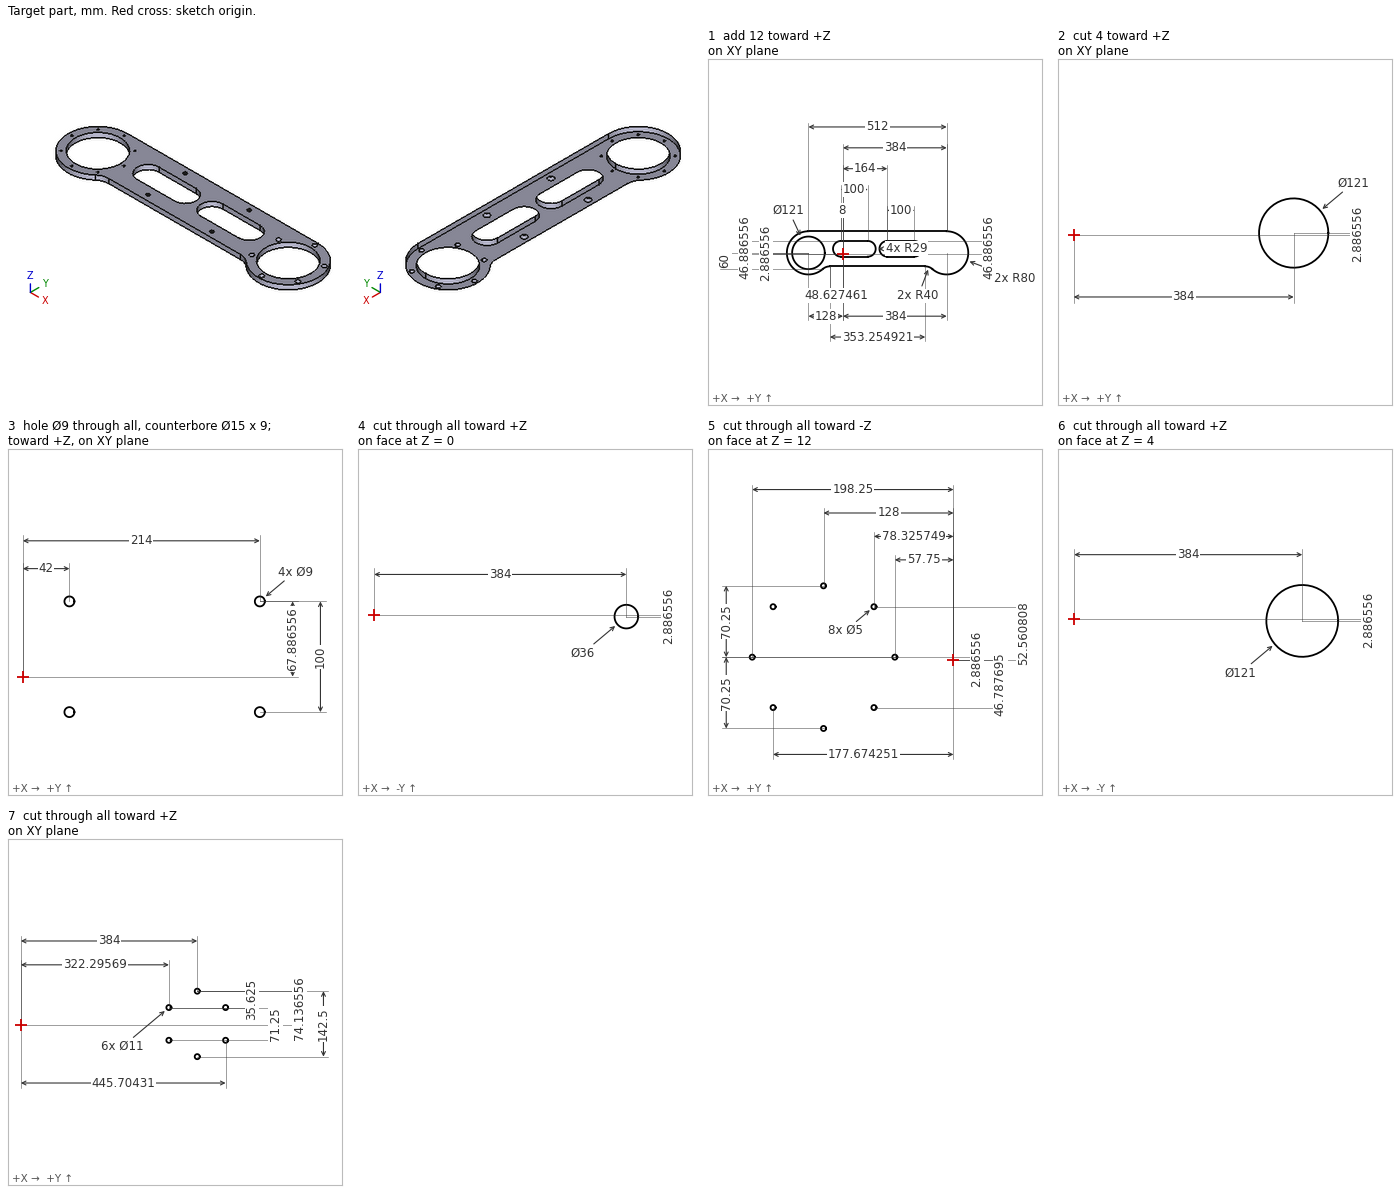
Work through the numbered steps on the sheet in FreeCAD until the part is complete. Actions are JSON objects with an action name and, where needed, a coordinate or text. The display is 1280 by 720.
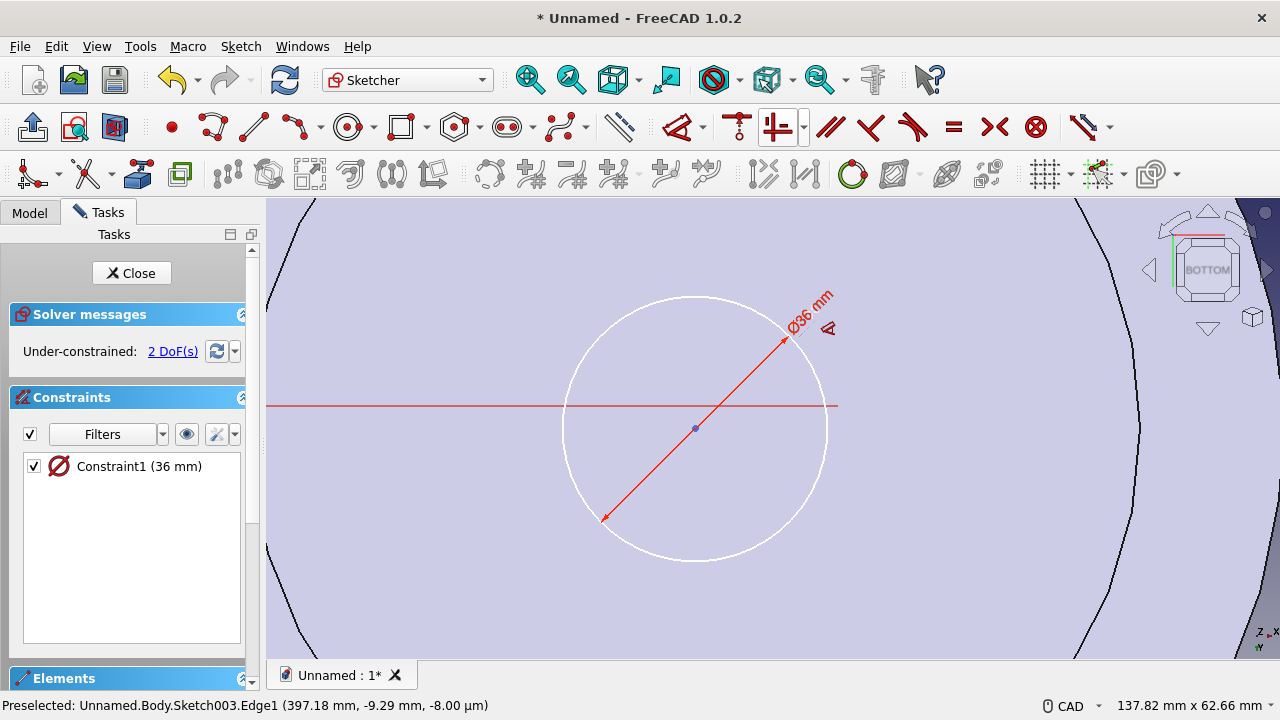
{"action": "left_click", "coordinate": [695, 429]}
{"action": "left_click", "coordinate": [495, 372]}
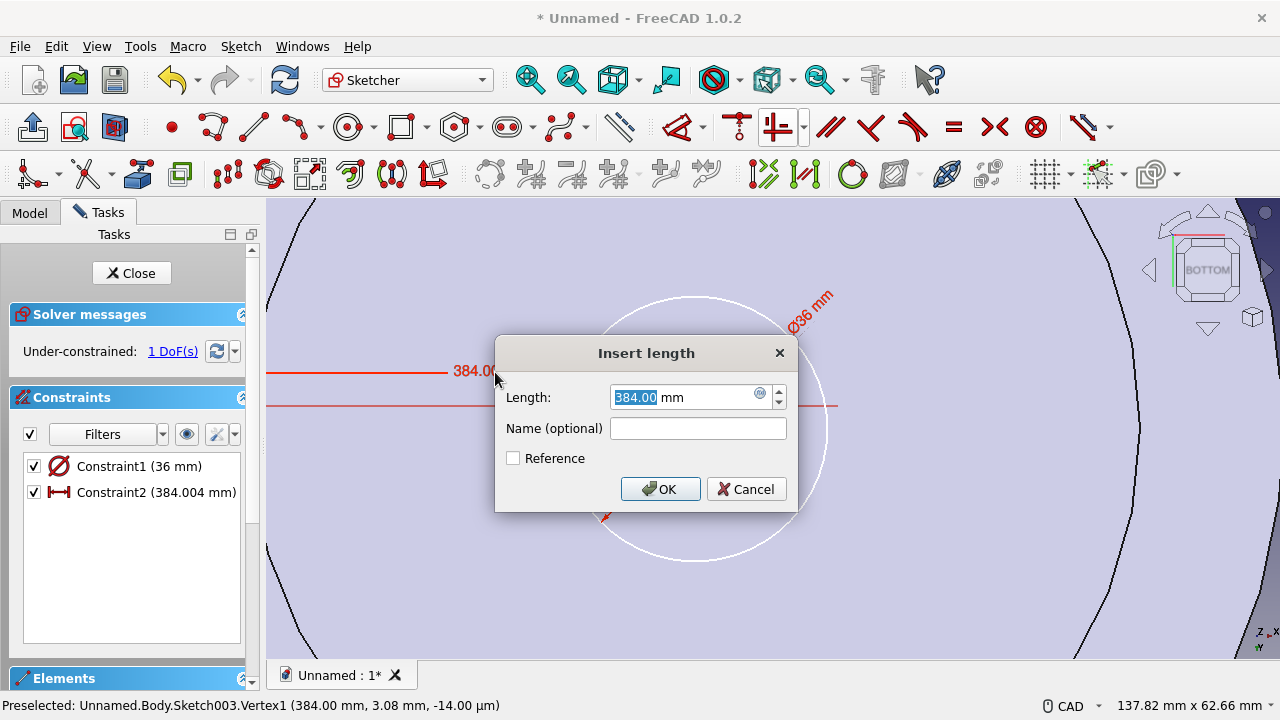
{"action": "type", "text": "384"}
{"action": "key", "text": "Return"}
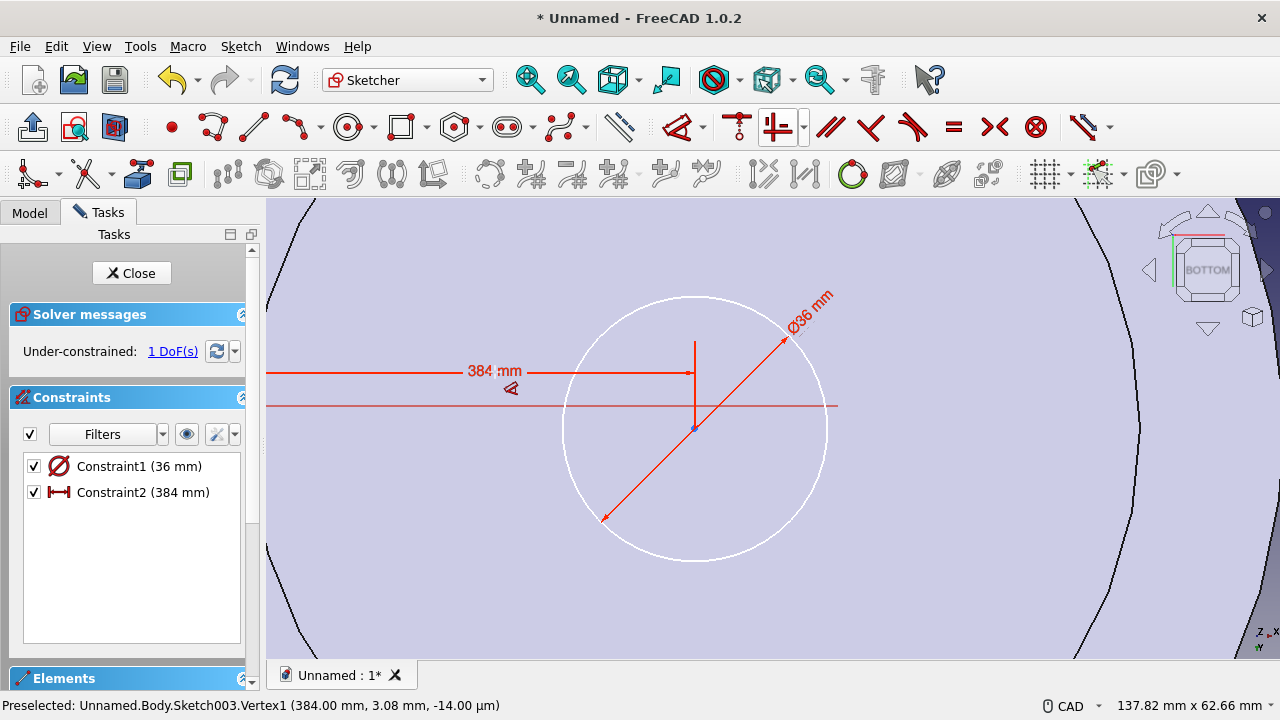
{"action": "scroll", "coordinate": [695, 429], "scroll_direction": "up", "scroll_amount": 4}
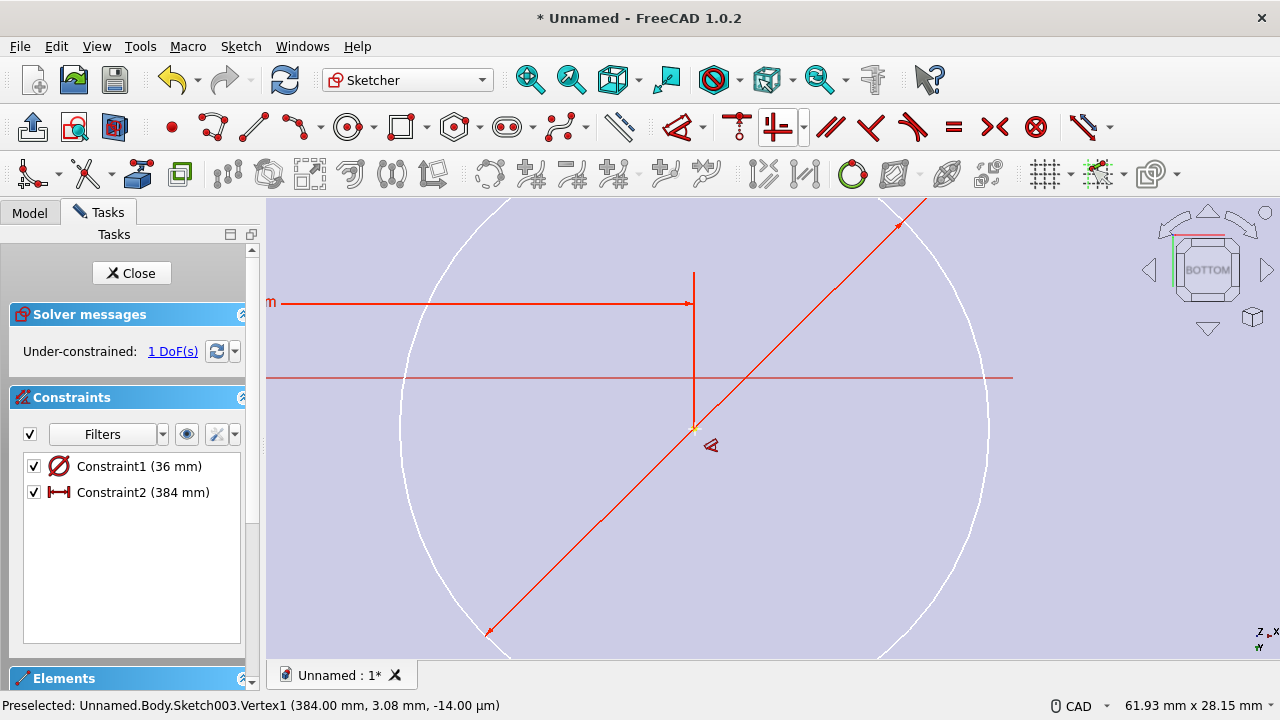
{"action": "left_click", "coordinate": [694, 428]}
{"action": "left_click", "coordinate": [728, 403]}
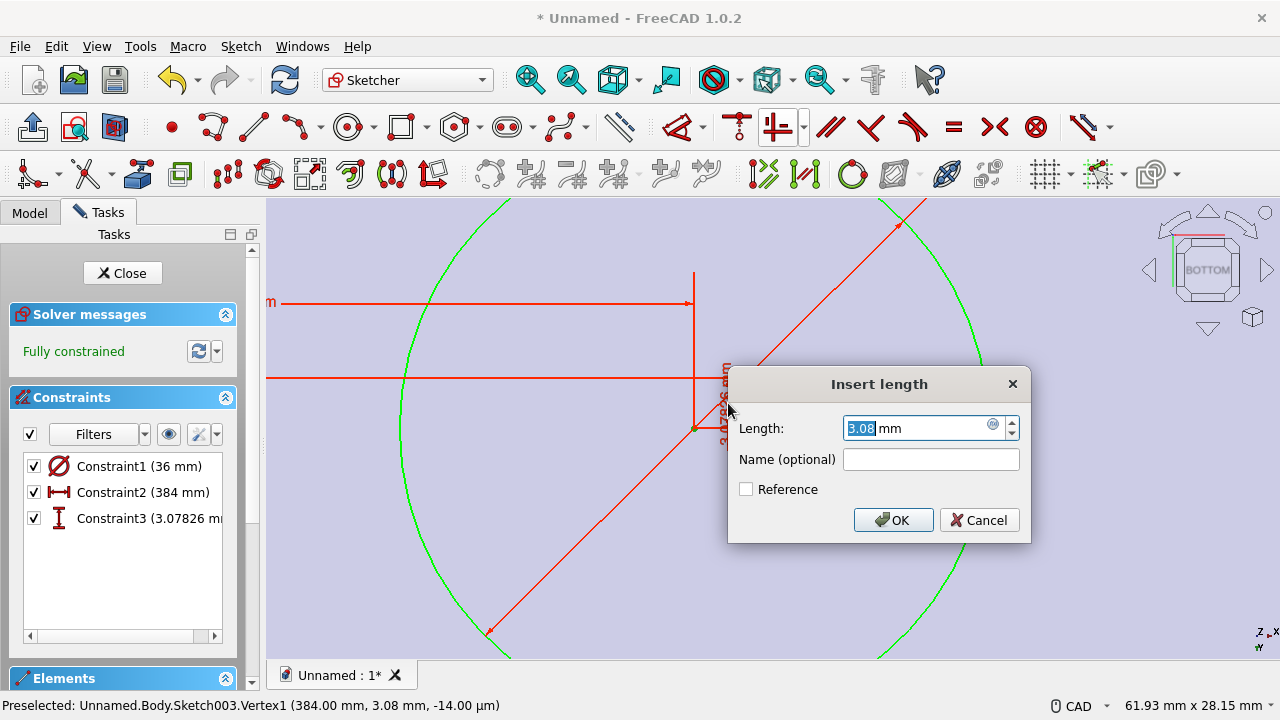
{"action": "type", "text": "2.886556"}
{"action": "key", "text": "Return"}
{"action": "key", "text": "Escape"}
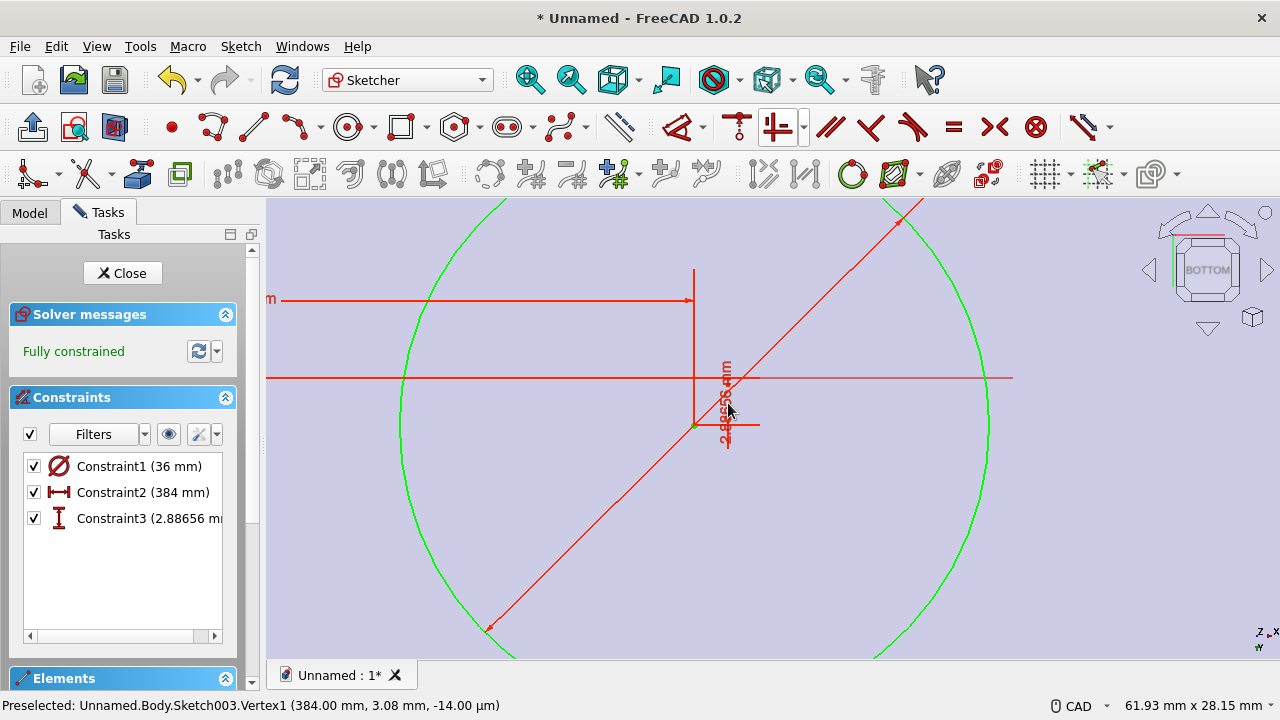
{"action": "left_click", "coordinate": [123, 273]}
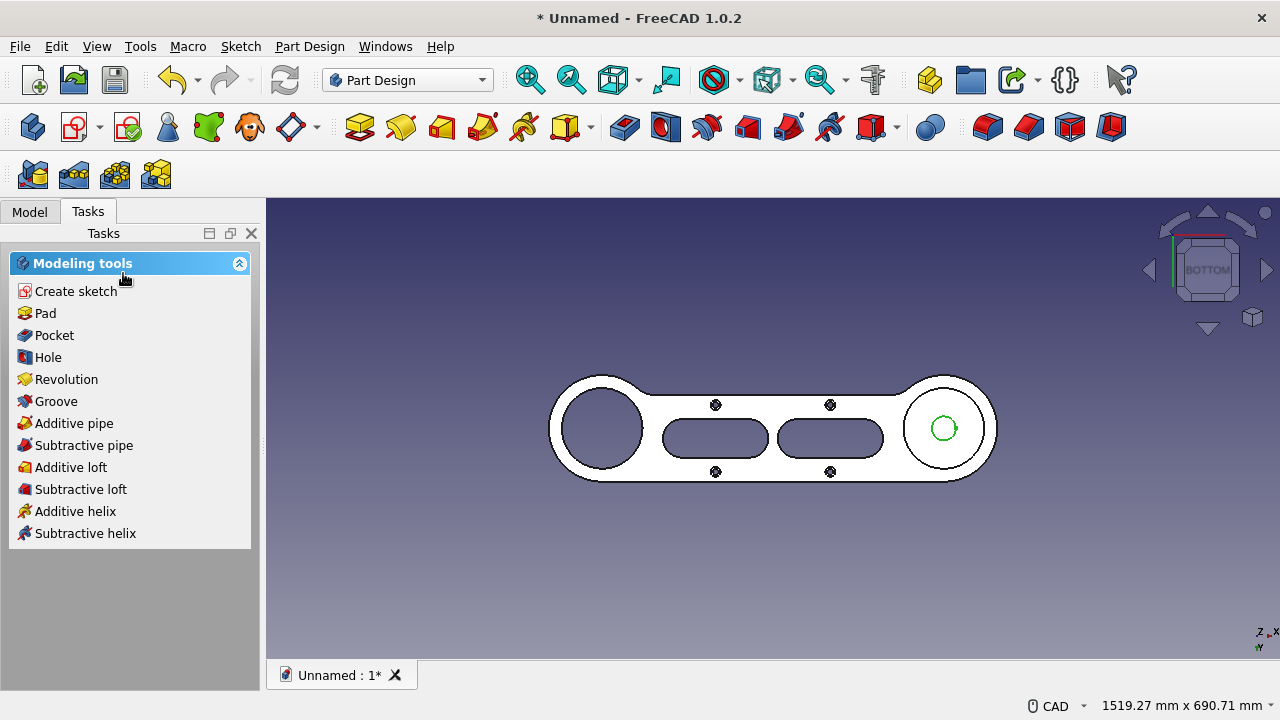
{"action": "left_click", "coordinate": [625, 128]}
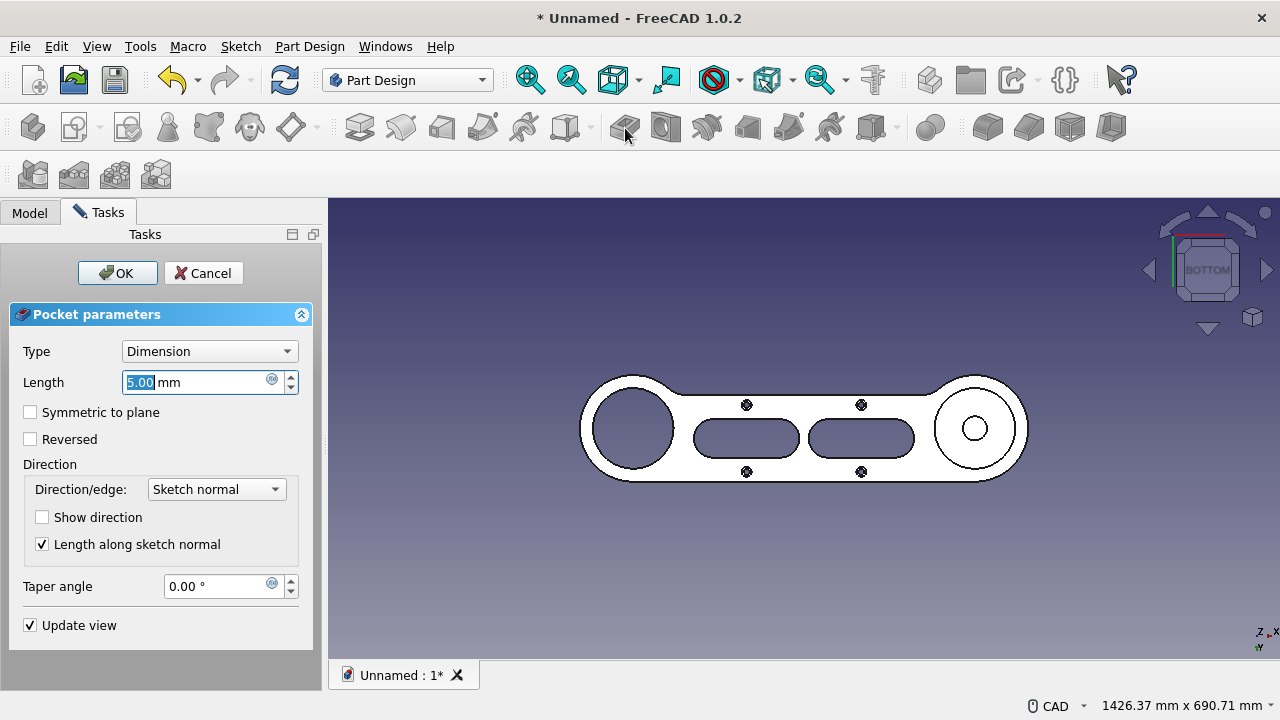
{"action": "left_click", "coordinate": [210, 352]}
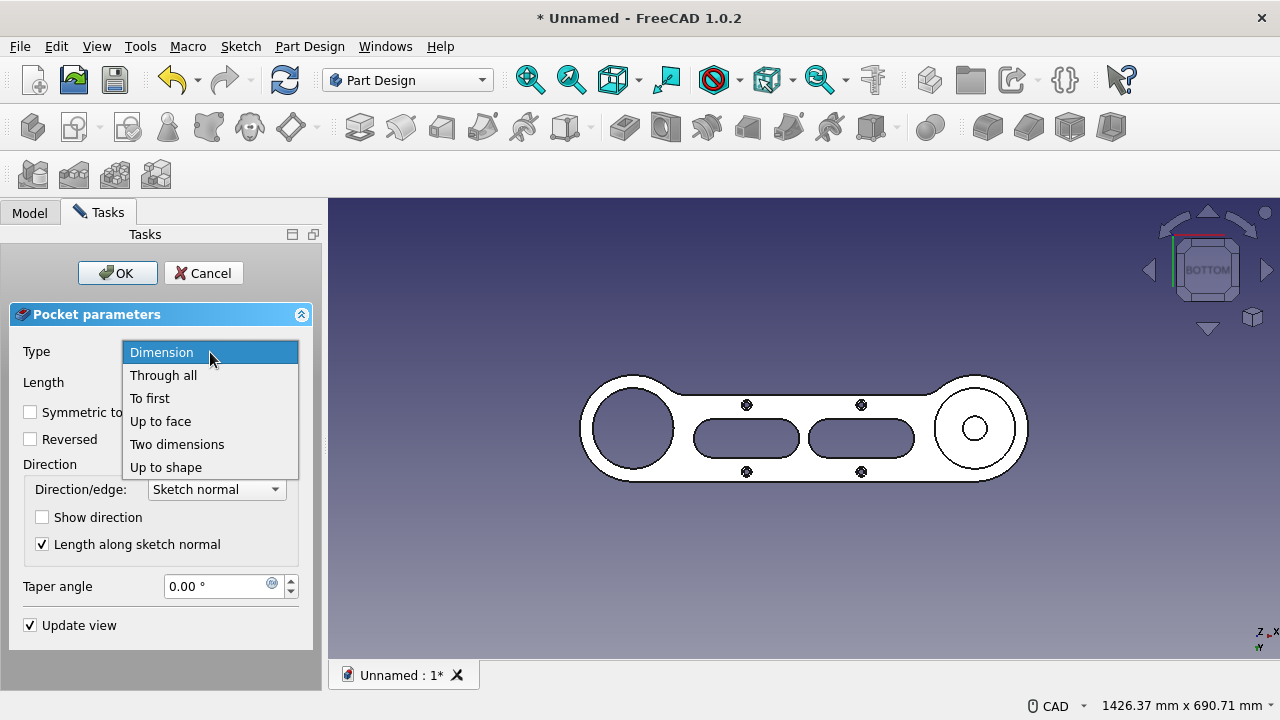
{"action": "left_click", "coordinate": [208, 376]}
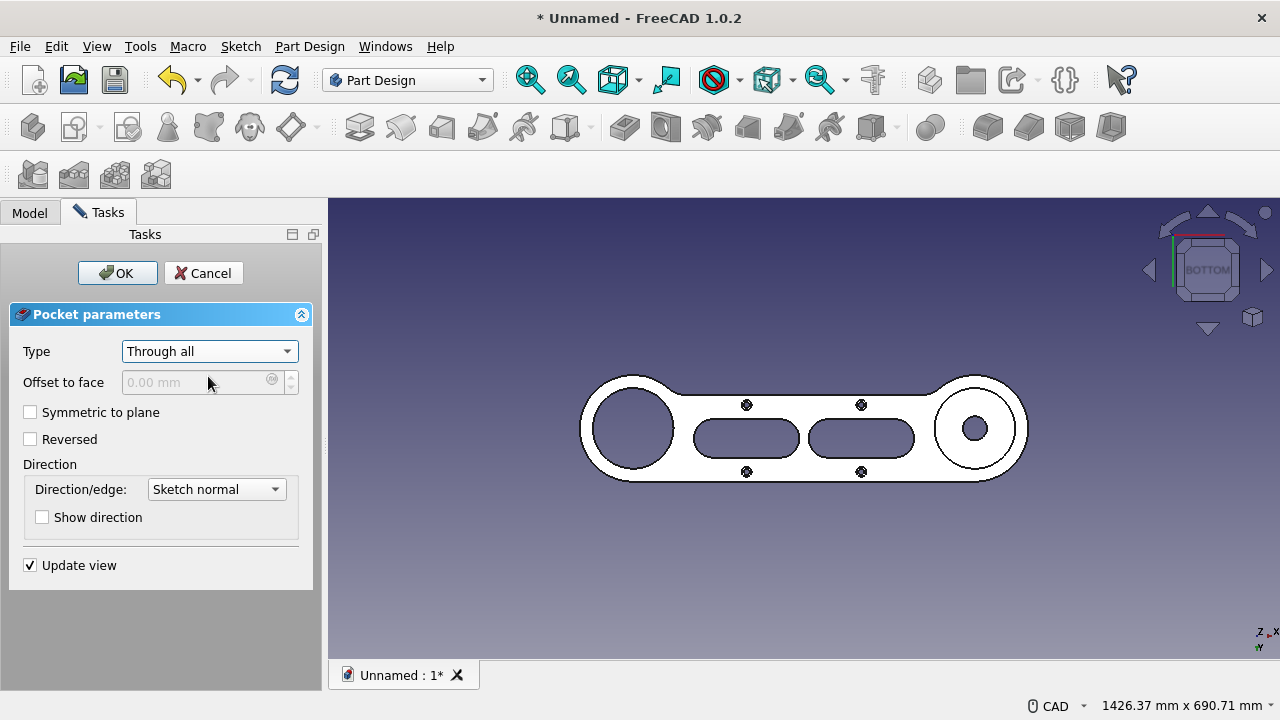
{"action": "left_click", "coordinate": [118, 273]}